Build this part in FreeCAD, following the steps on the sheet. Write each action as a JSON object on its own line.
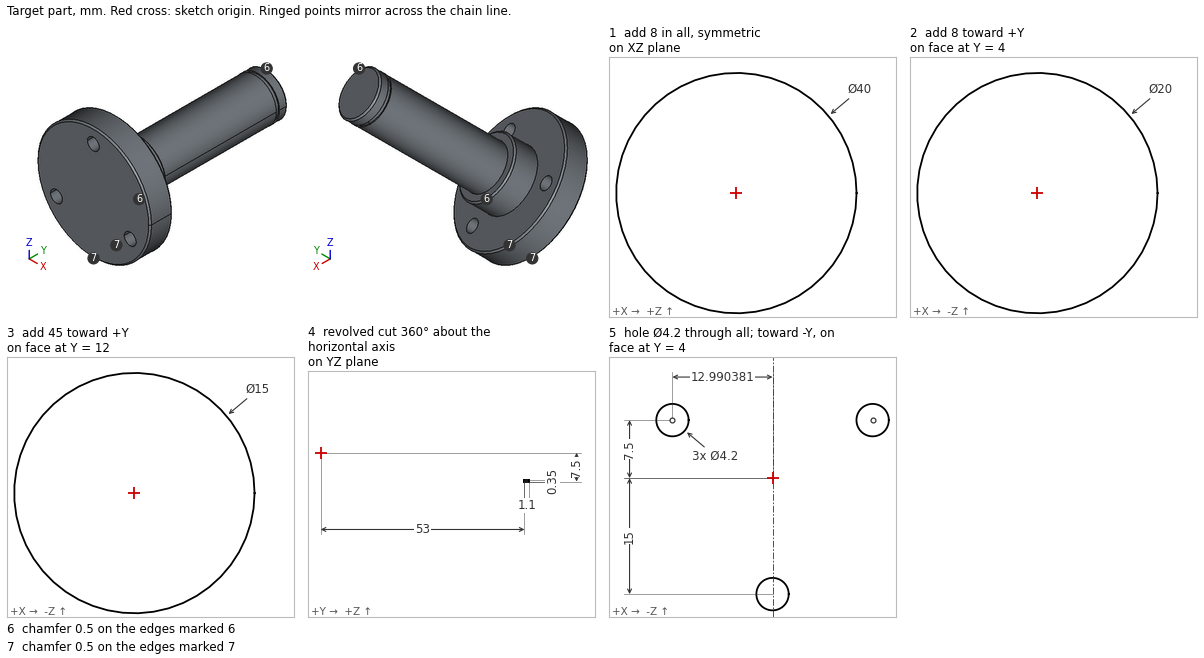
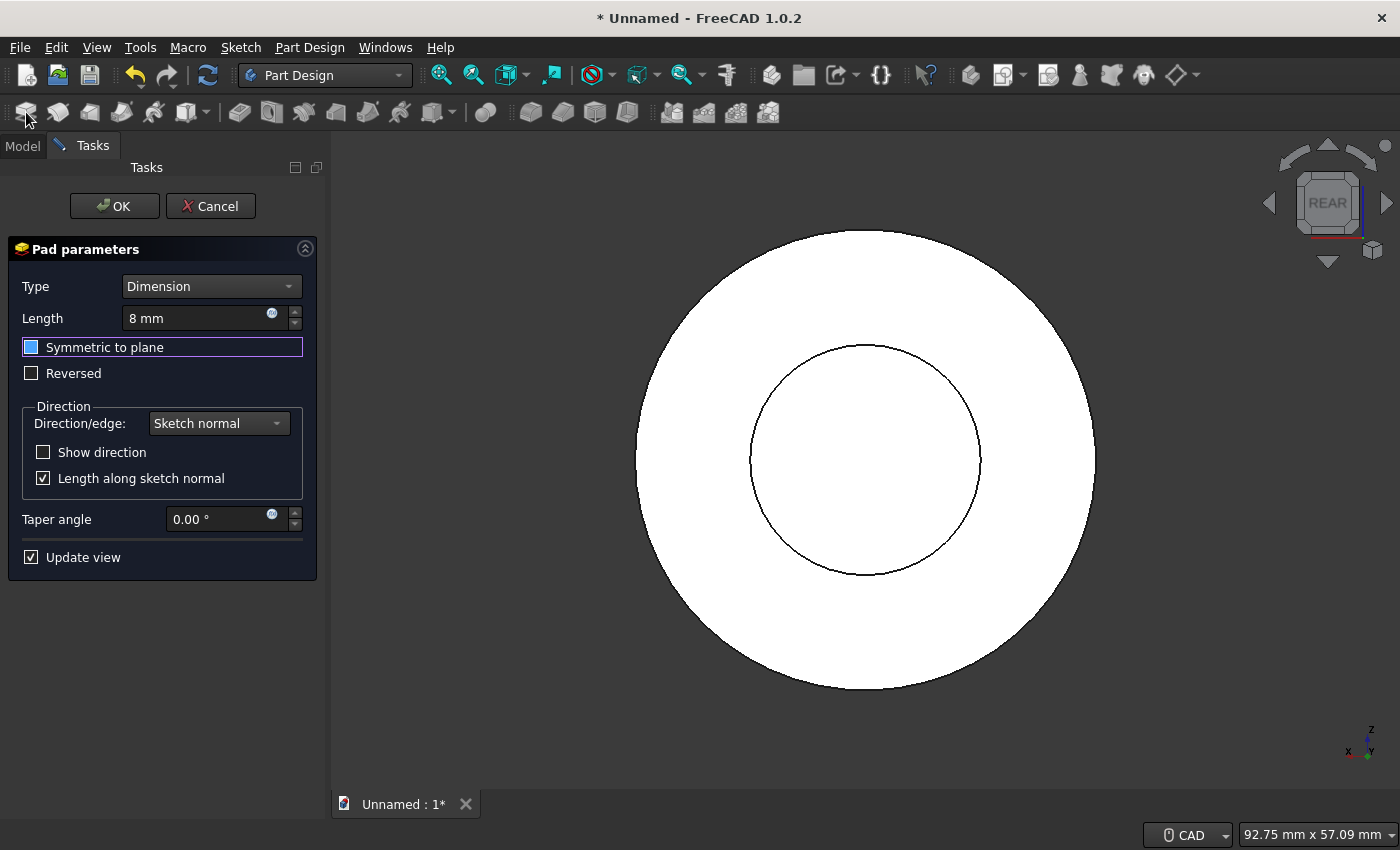
{"action": "left_click", "coordinate": [115, 206]}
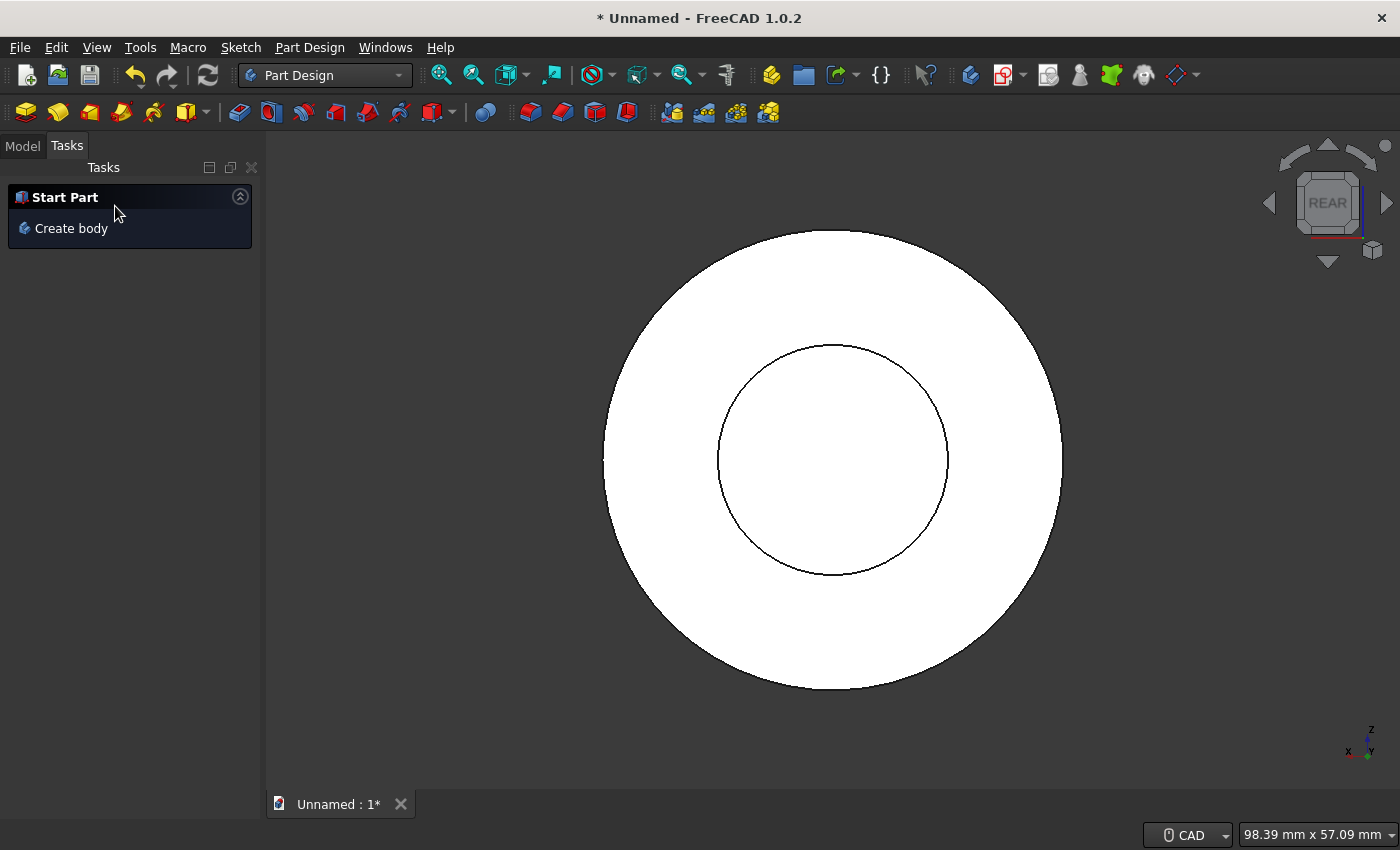
{"action": "left_click", "coordinate": [833, 459]}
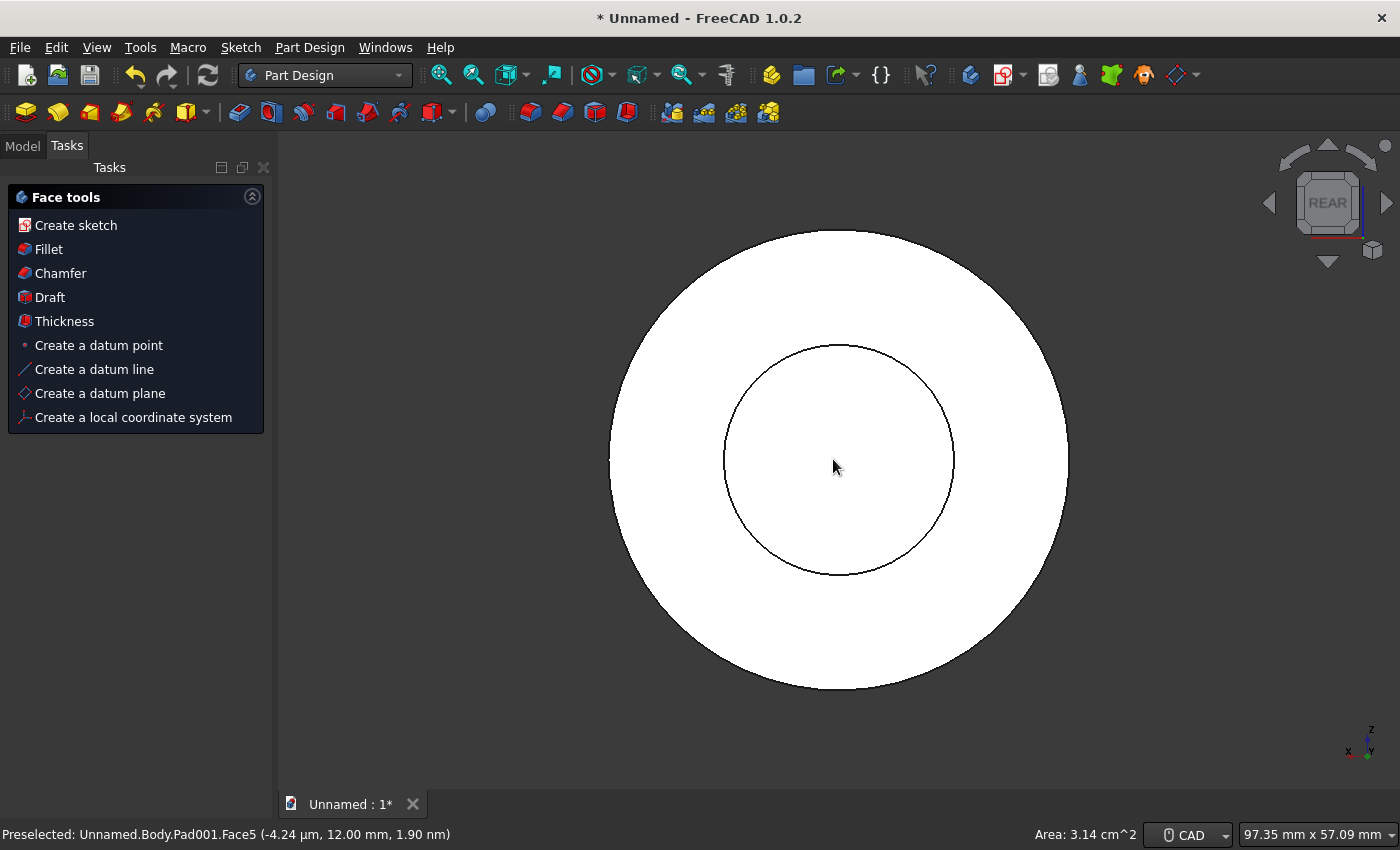
{"action": "left_click", "coordinate": [1004, 76]}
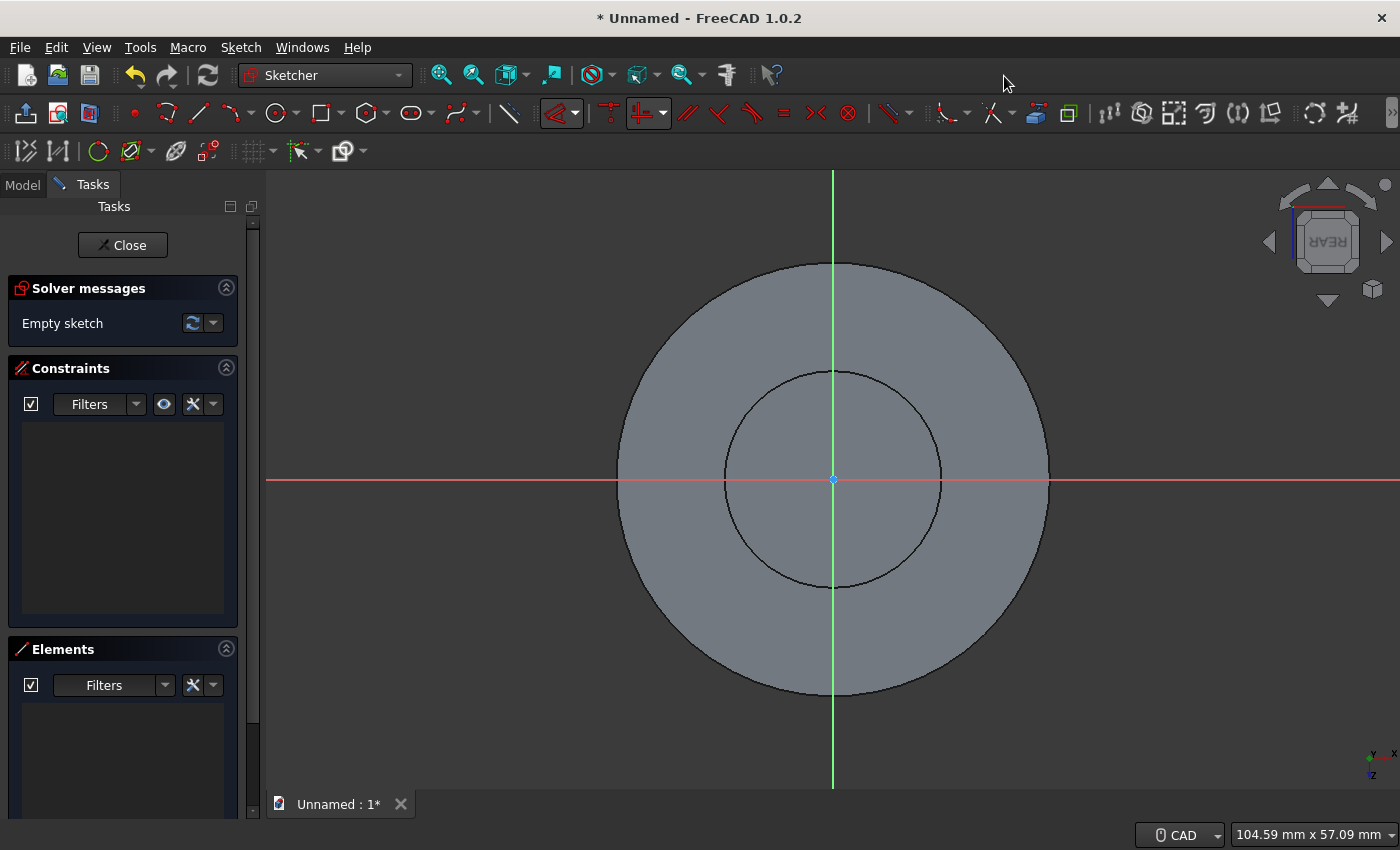
{"action": "scroll", "coordinate": [889, 479], "scroll_direction": "up", "scroll_amount": 4}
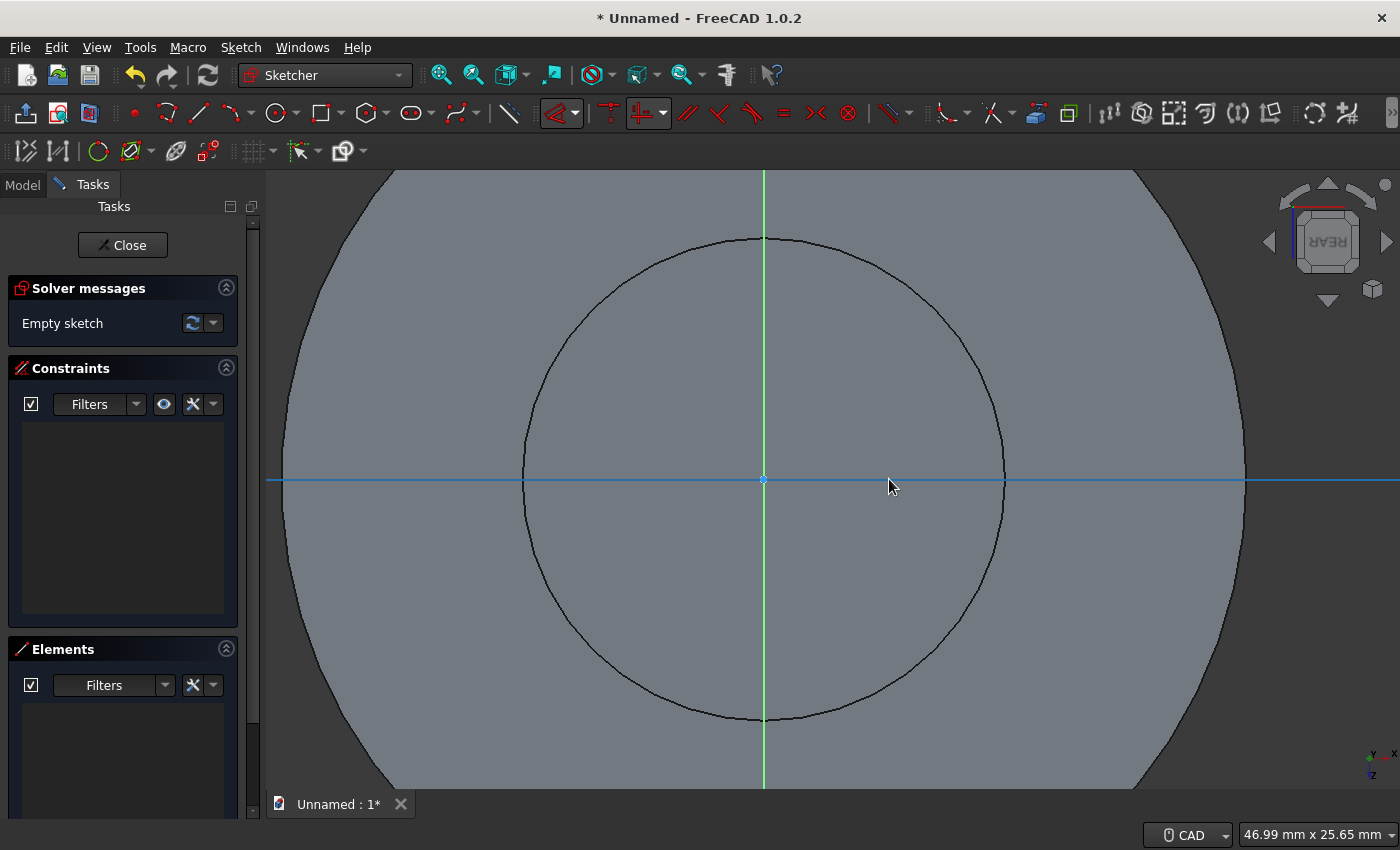
{"action": "left_click", "coordinate": [276, 114]}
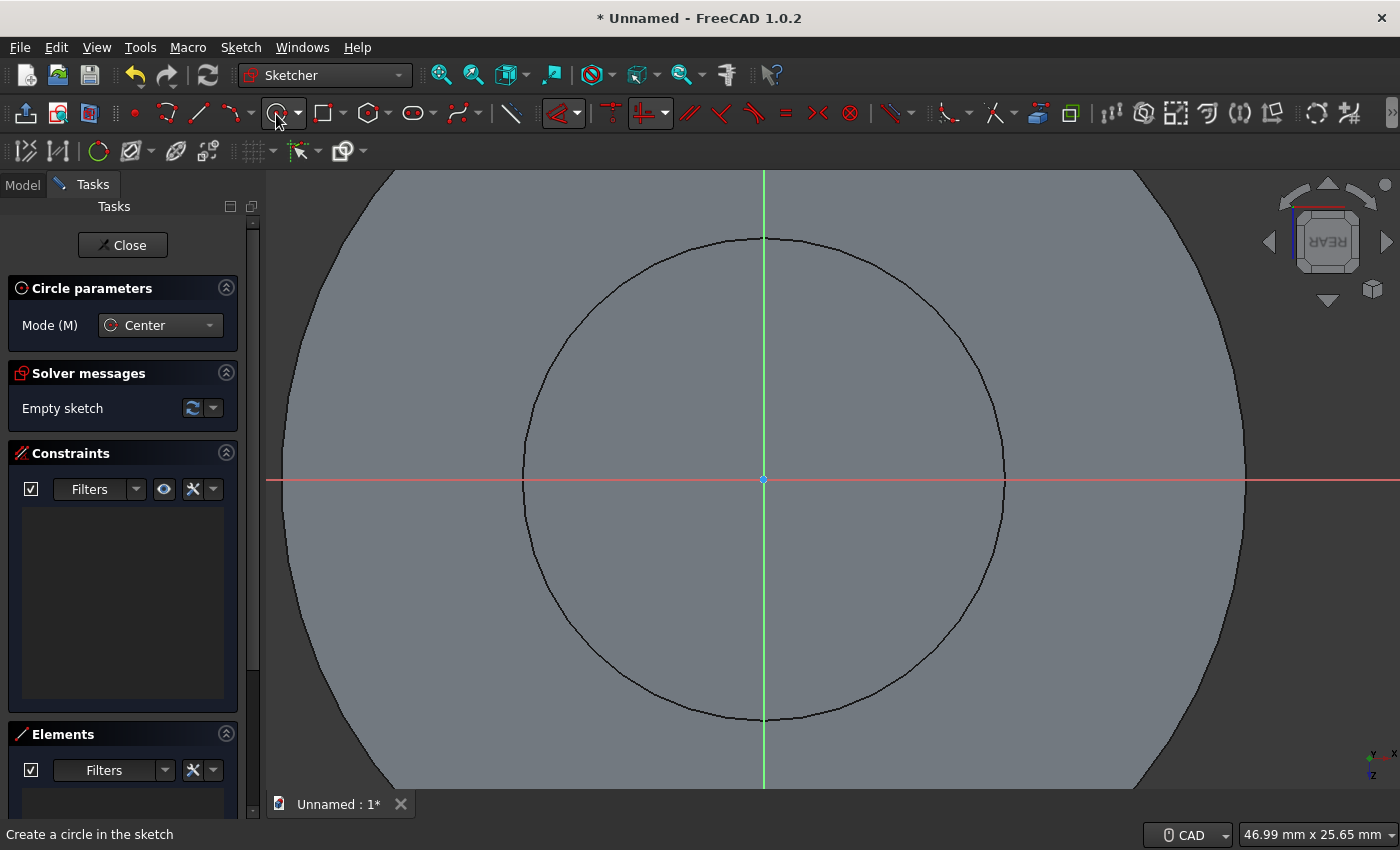
{"action": "left_click", "coordinate": [764, 479]}
{"action": "mouse_move", "coordinate": [892, 352]}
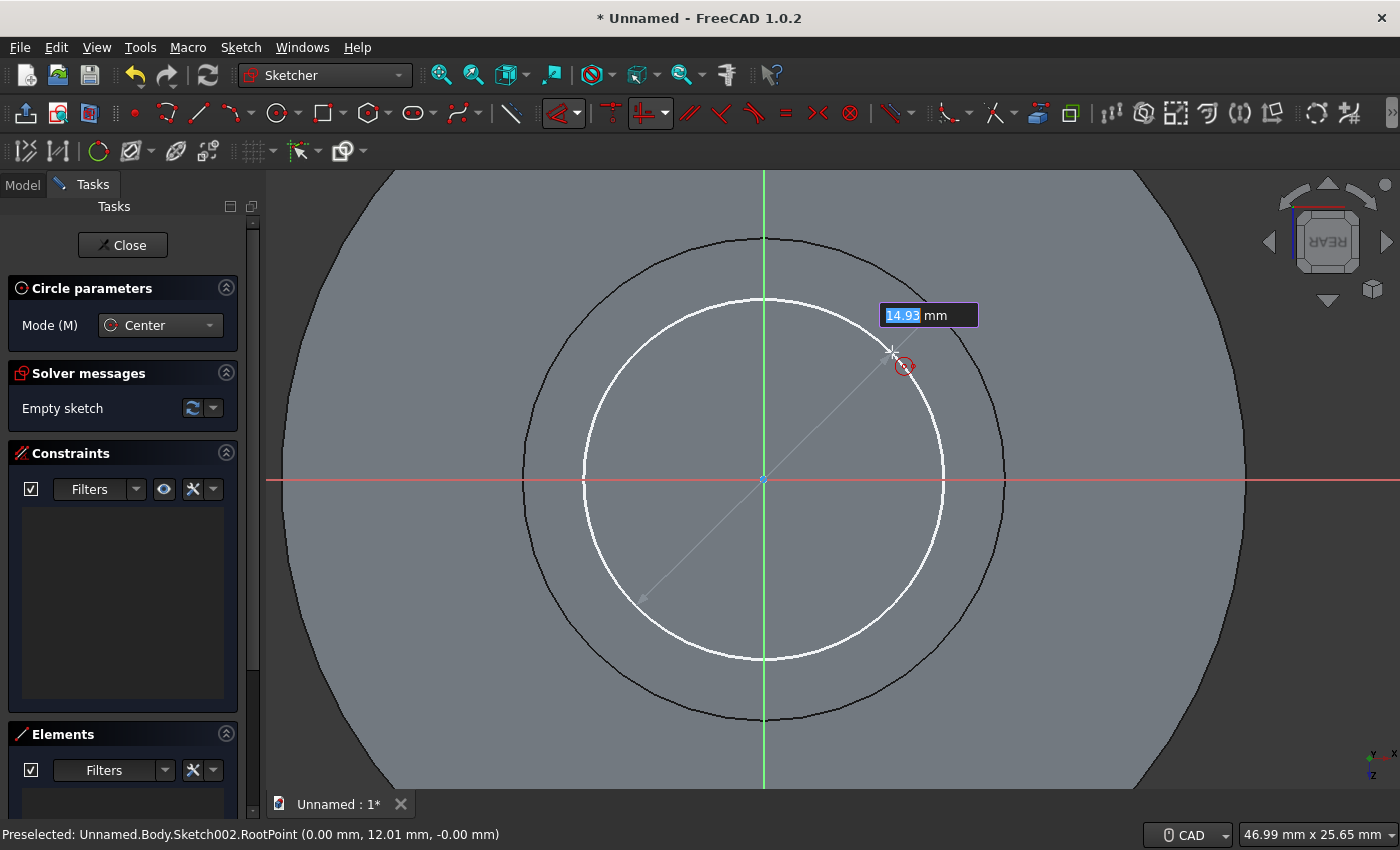
{"action": "type", "text": "15"}
{"action": "key", "text": "Return"}
{"action": "key", "text": "Escape"}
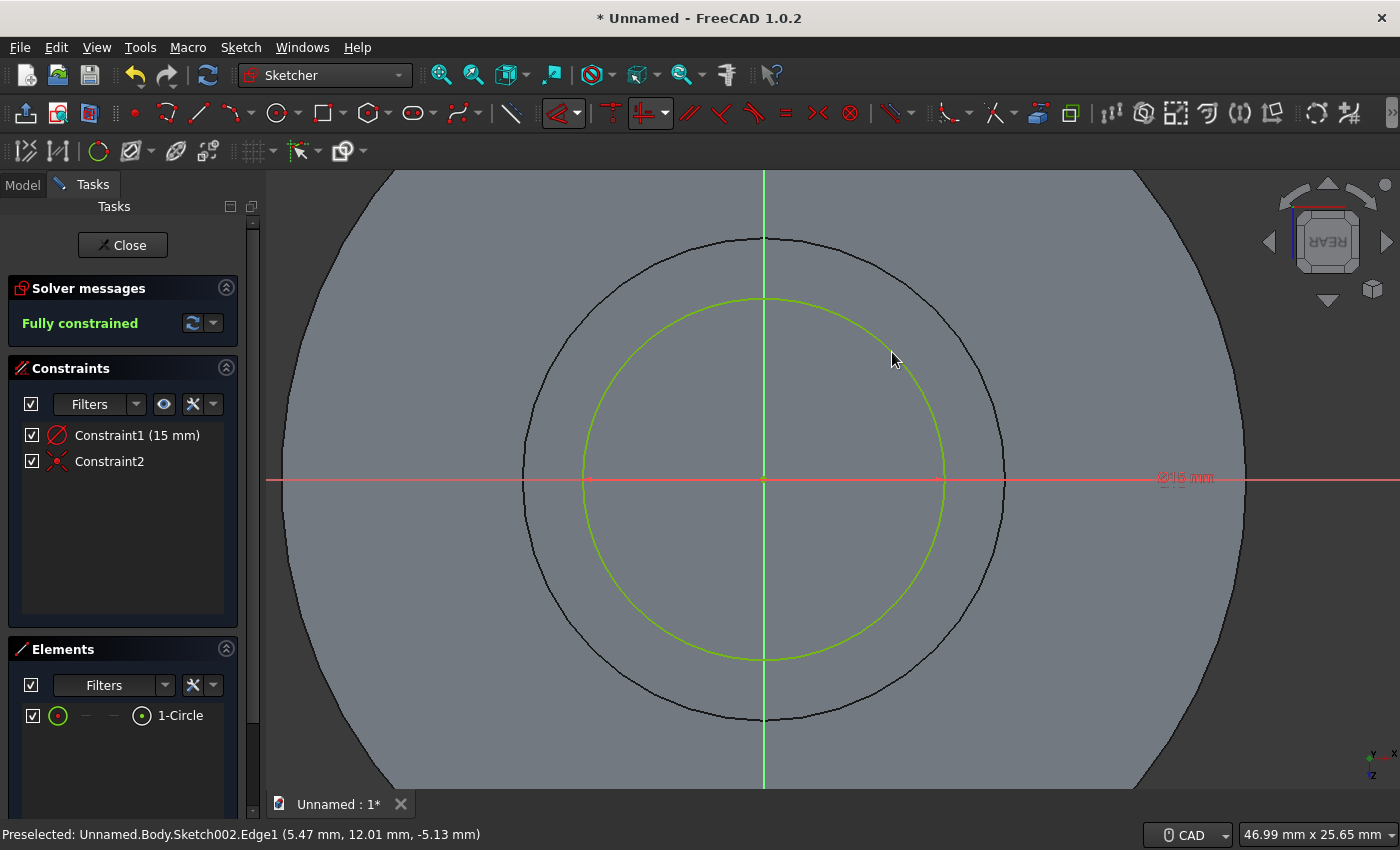
{"action": "left_click", "coordinate": [123, 245]}